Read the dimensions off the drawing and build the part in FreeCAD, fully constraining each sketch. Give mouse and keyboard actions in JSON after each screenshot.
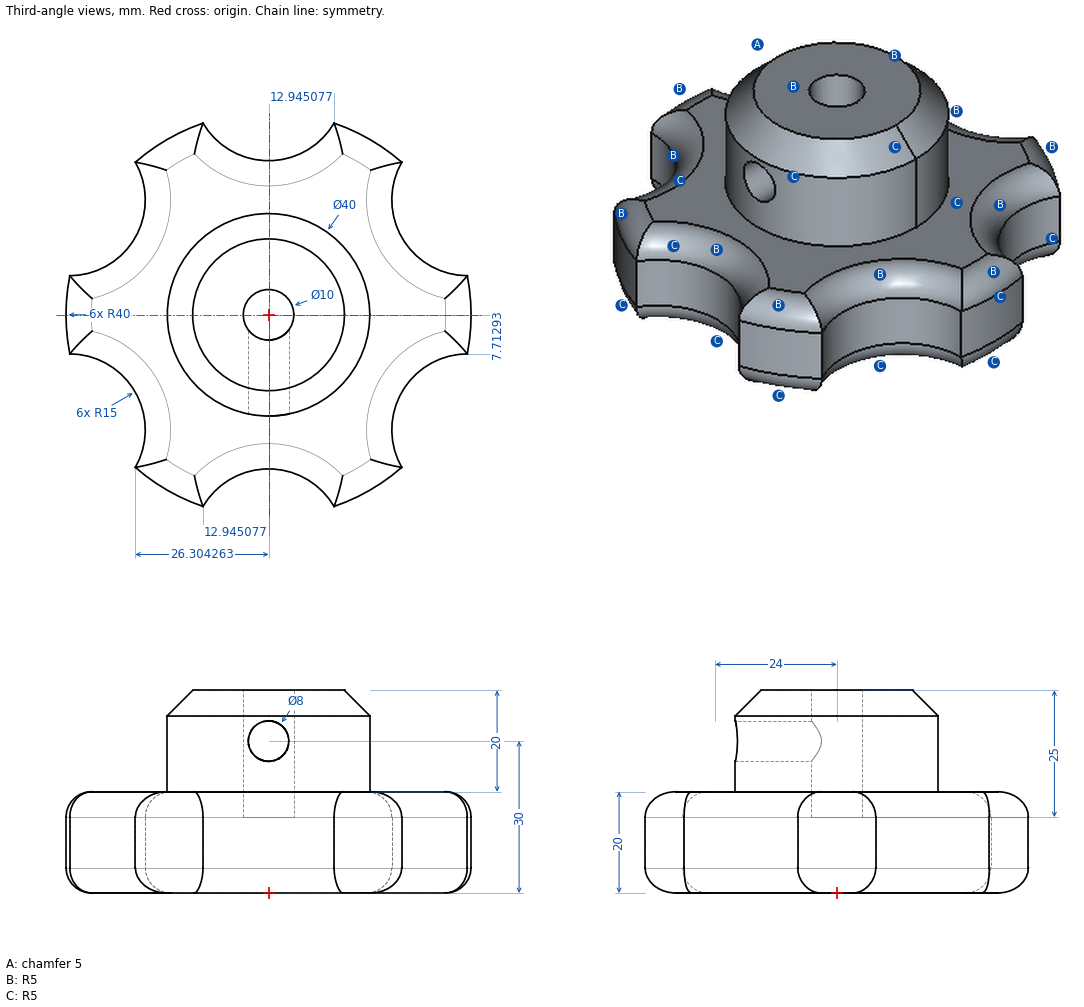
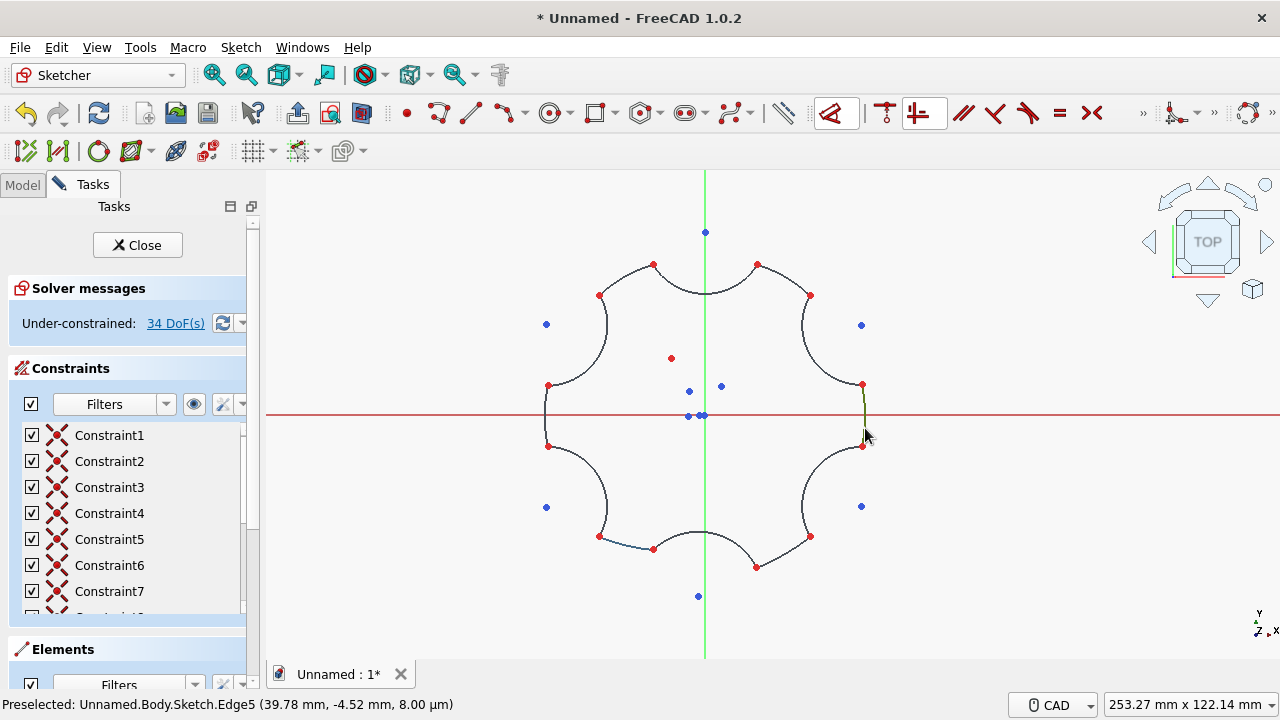
{"action": "left_click", "coordinate": [886, 114]}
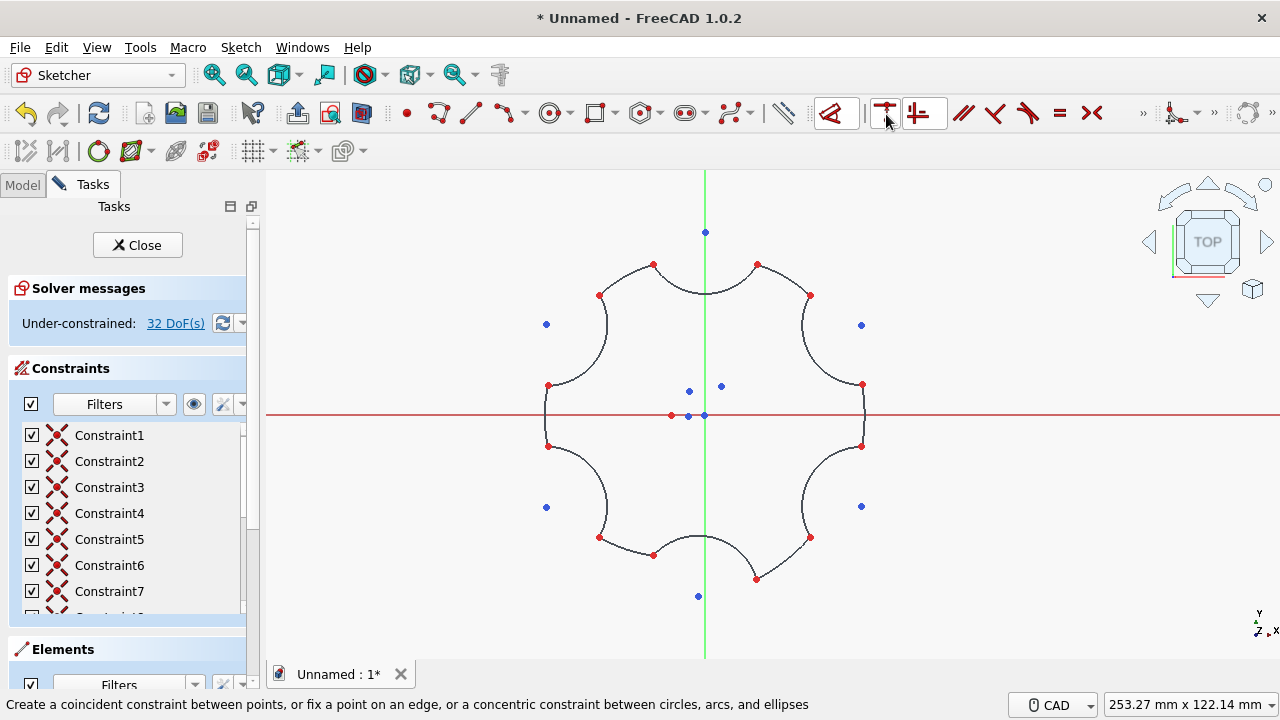
{"action": "left_click", "coordinate": [614, 545]}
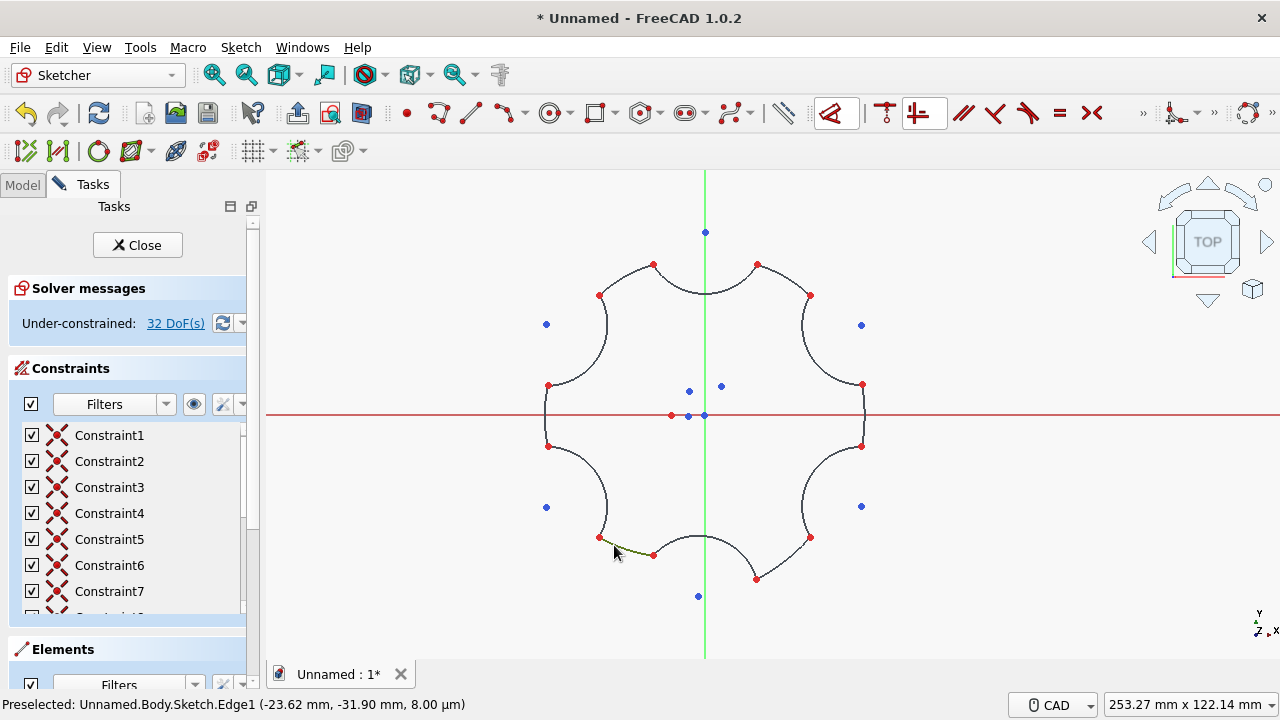
{"action": "left_click", "coordinate": [796, 284]}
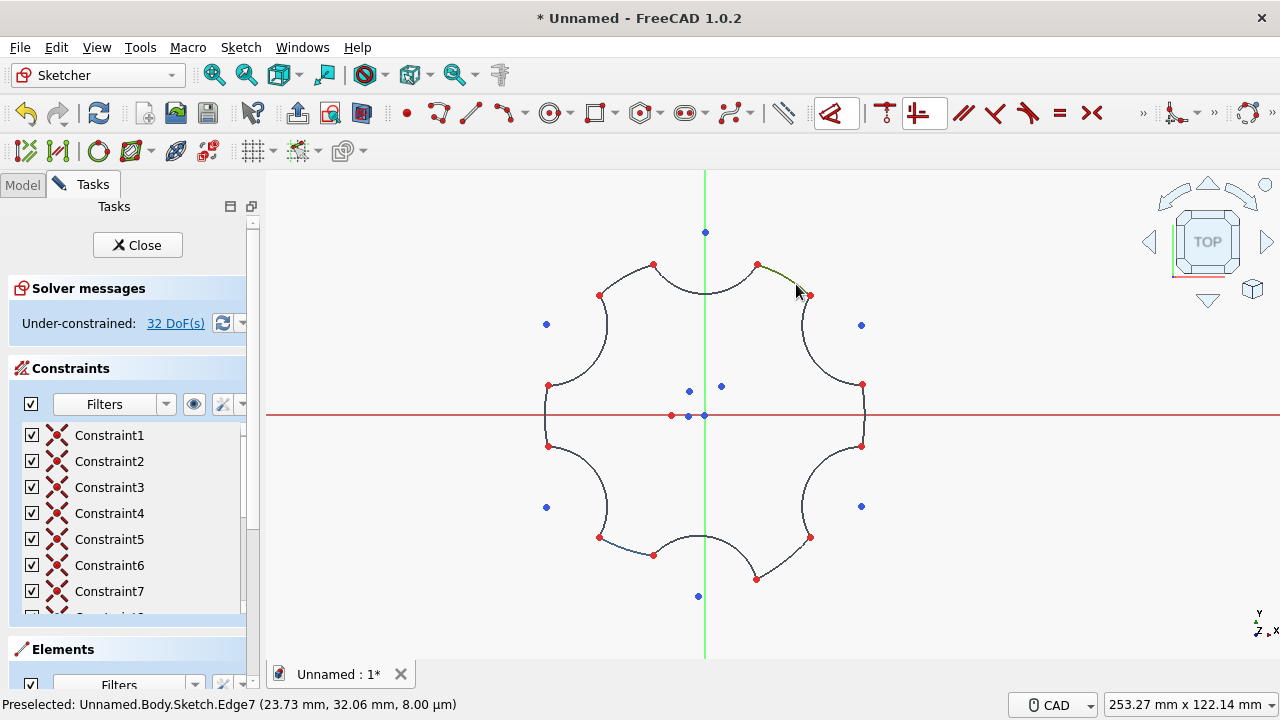
{"action": "left_click", "coordinate": [886, 114]}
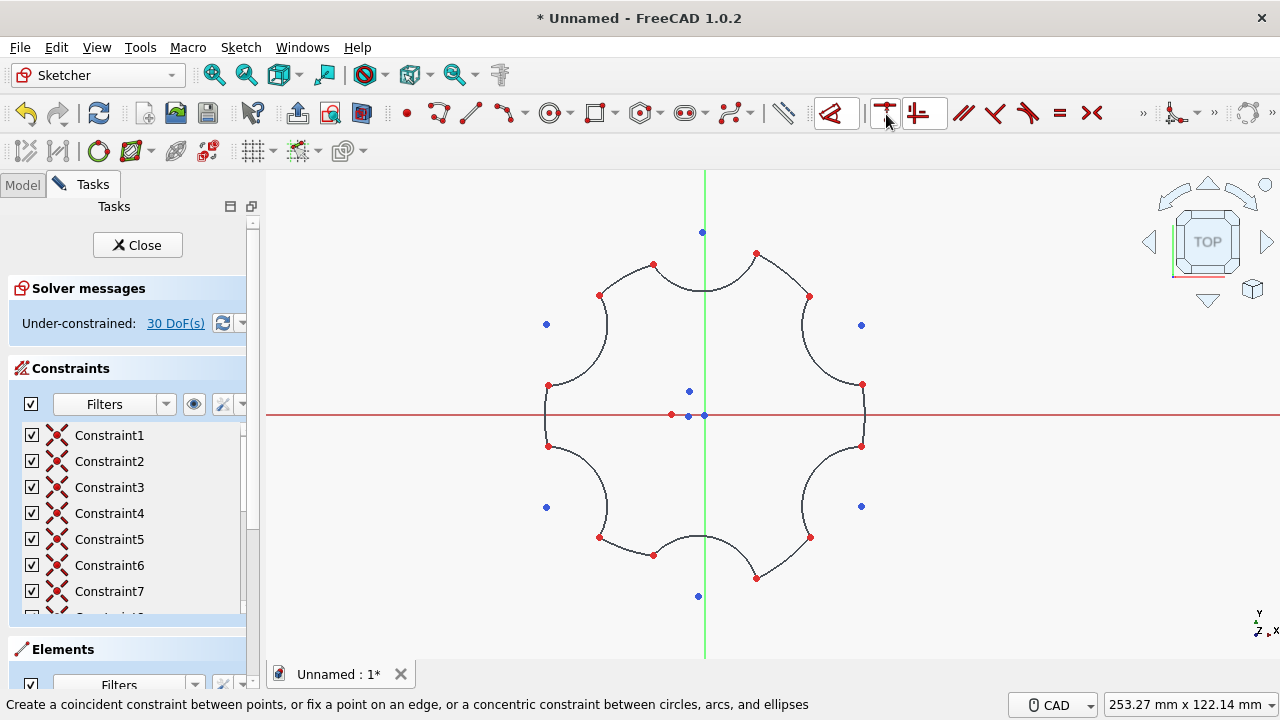
{"action": "left_click", "coordinate": [614, 545]}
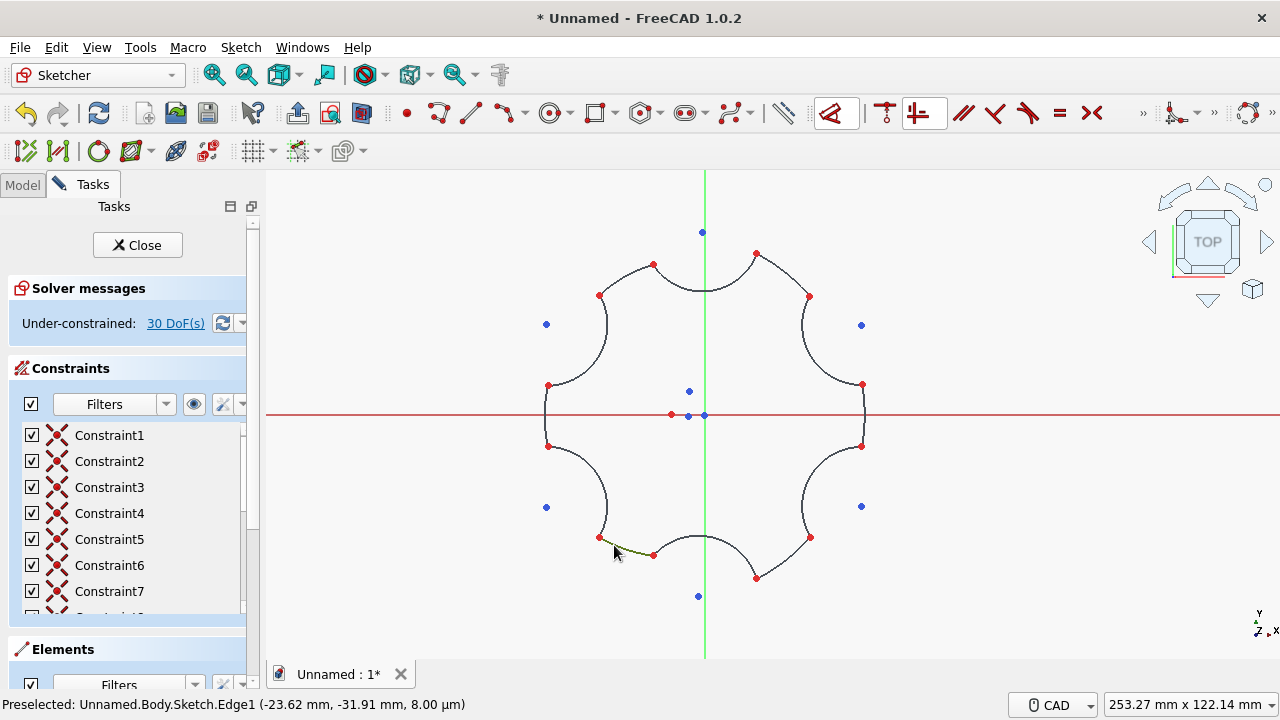
{"action": "left_click", "coordinate": [636, 271]}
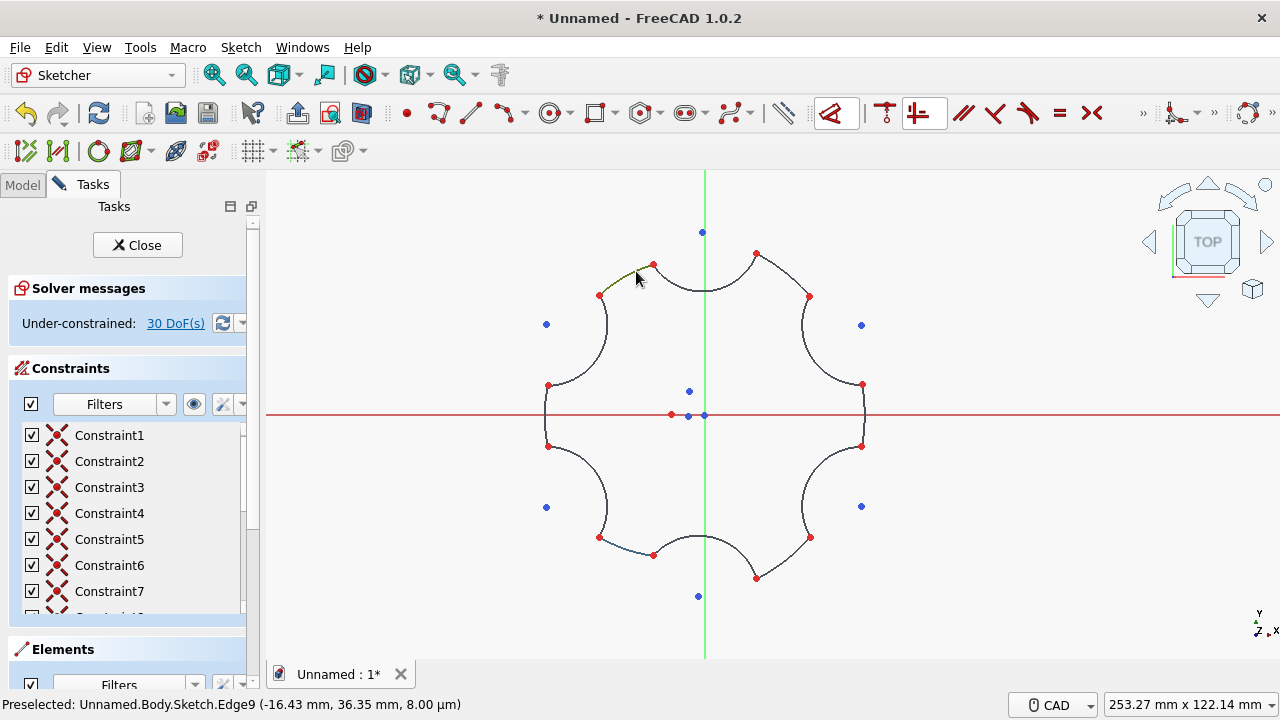
{"action": "left_click", "coordinate": [886, 114]}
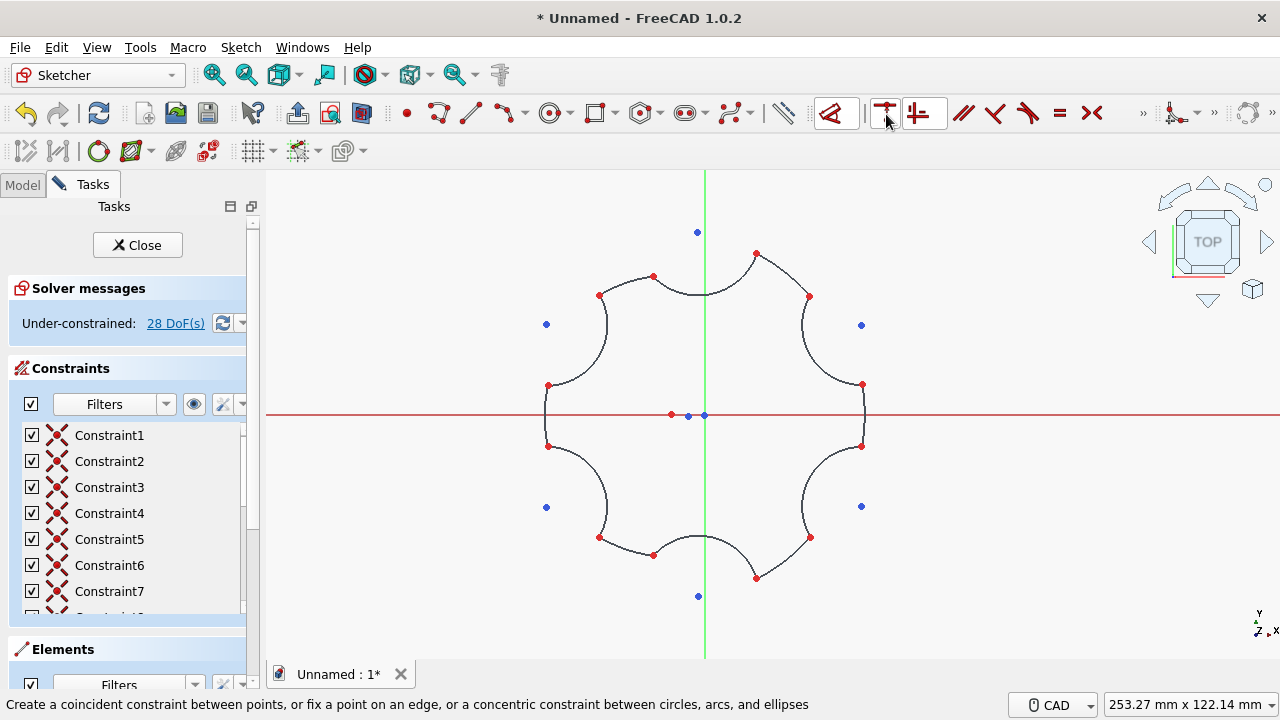
{"action": "left_click", "coordinate": [614, 545]}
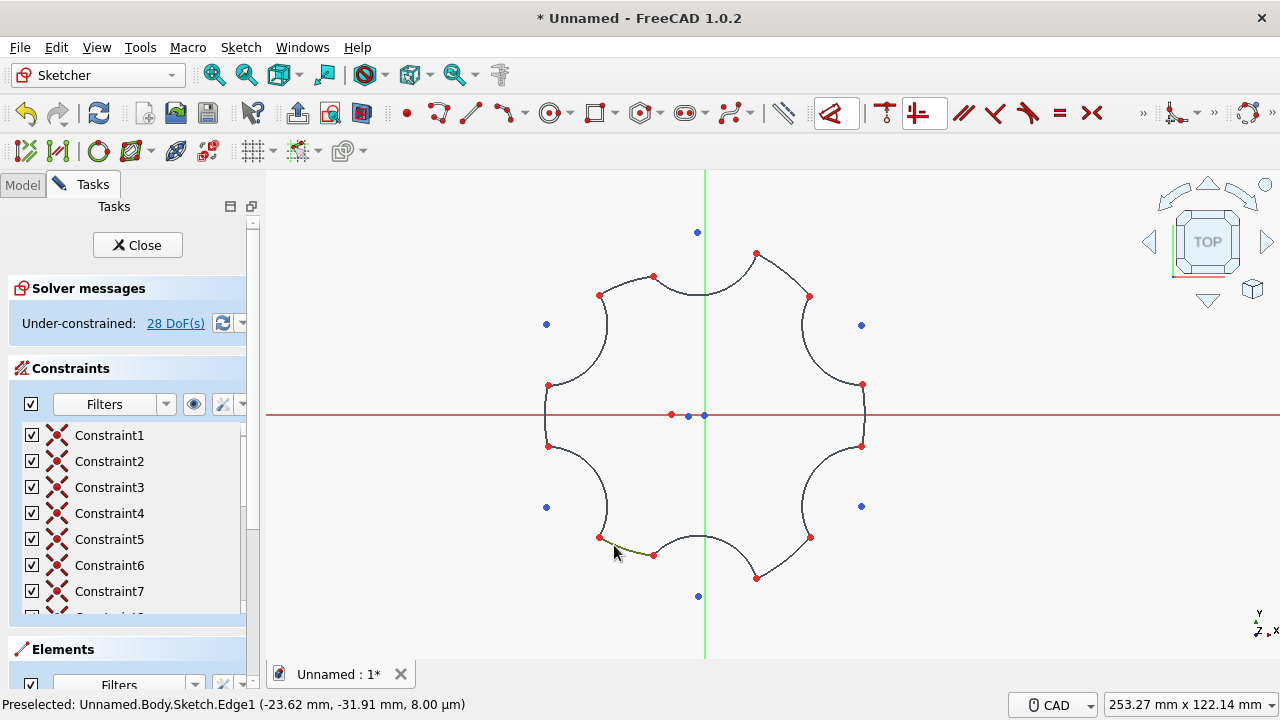
{"action": "scroll", "coordinate": [545, 404], "scroll_direction": "up", "scroll_amount": 2}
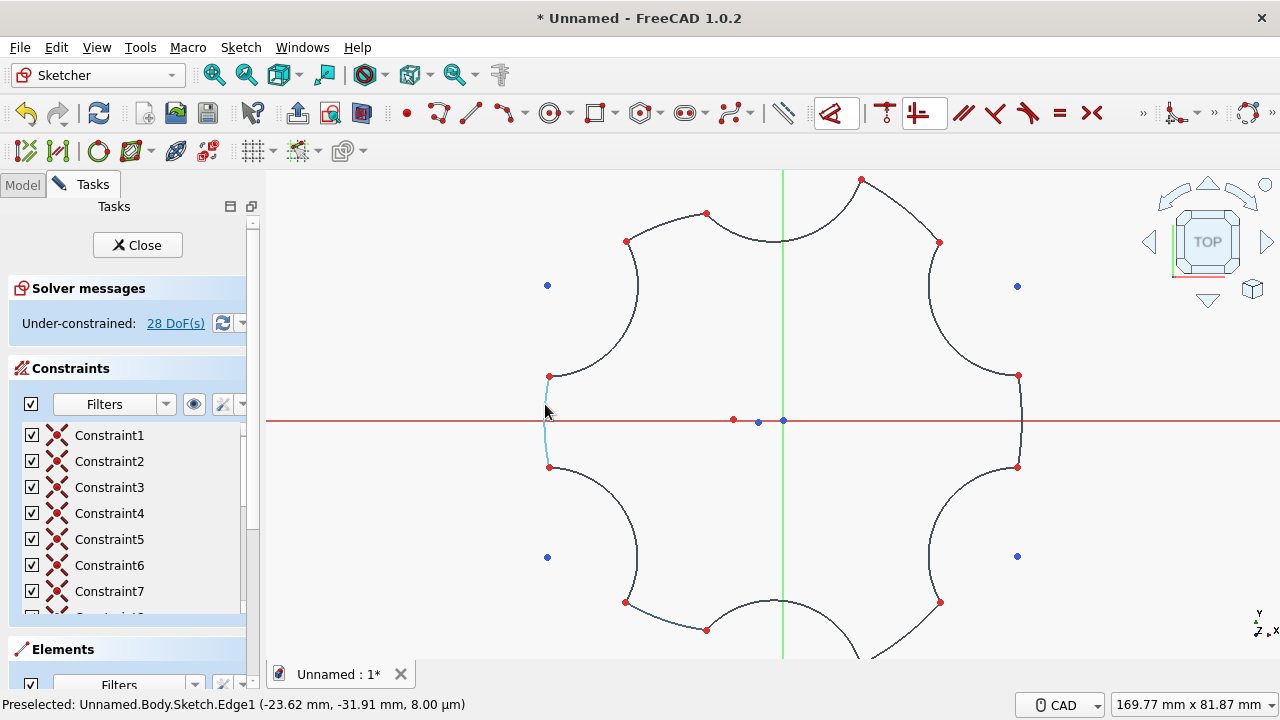
{"action": "left_click", "coordinate": [545, 404]}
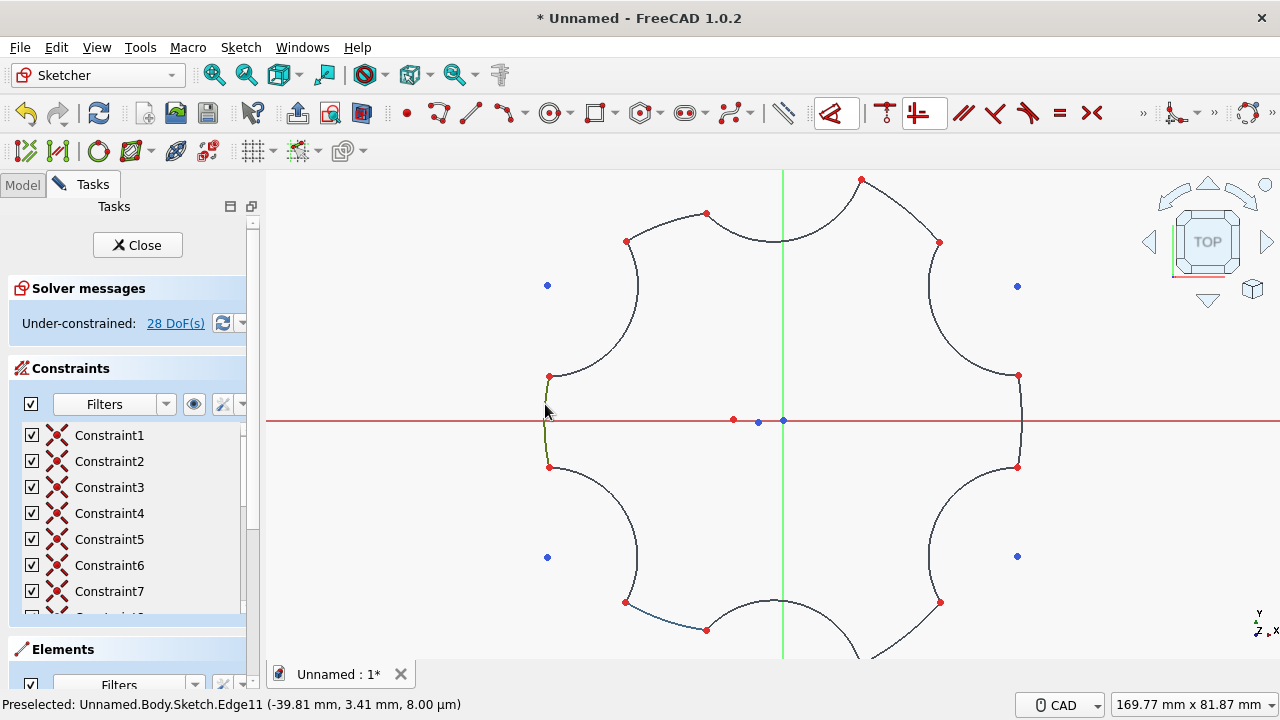
{"action": "left_click", "coordinate": [886, 114]}